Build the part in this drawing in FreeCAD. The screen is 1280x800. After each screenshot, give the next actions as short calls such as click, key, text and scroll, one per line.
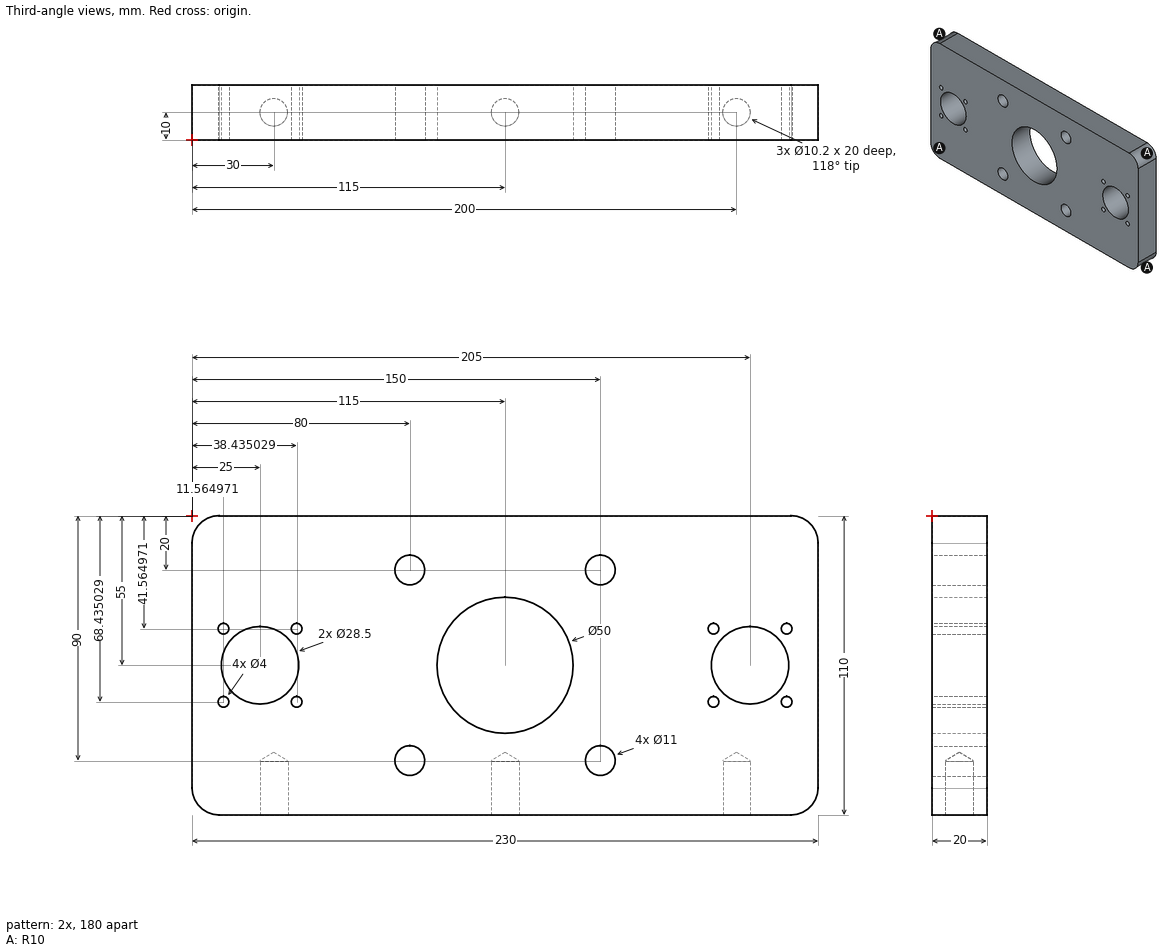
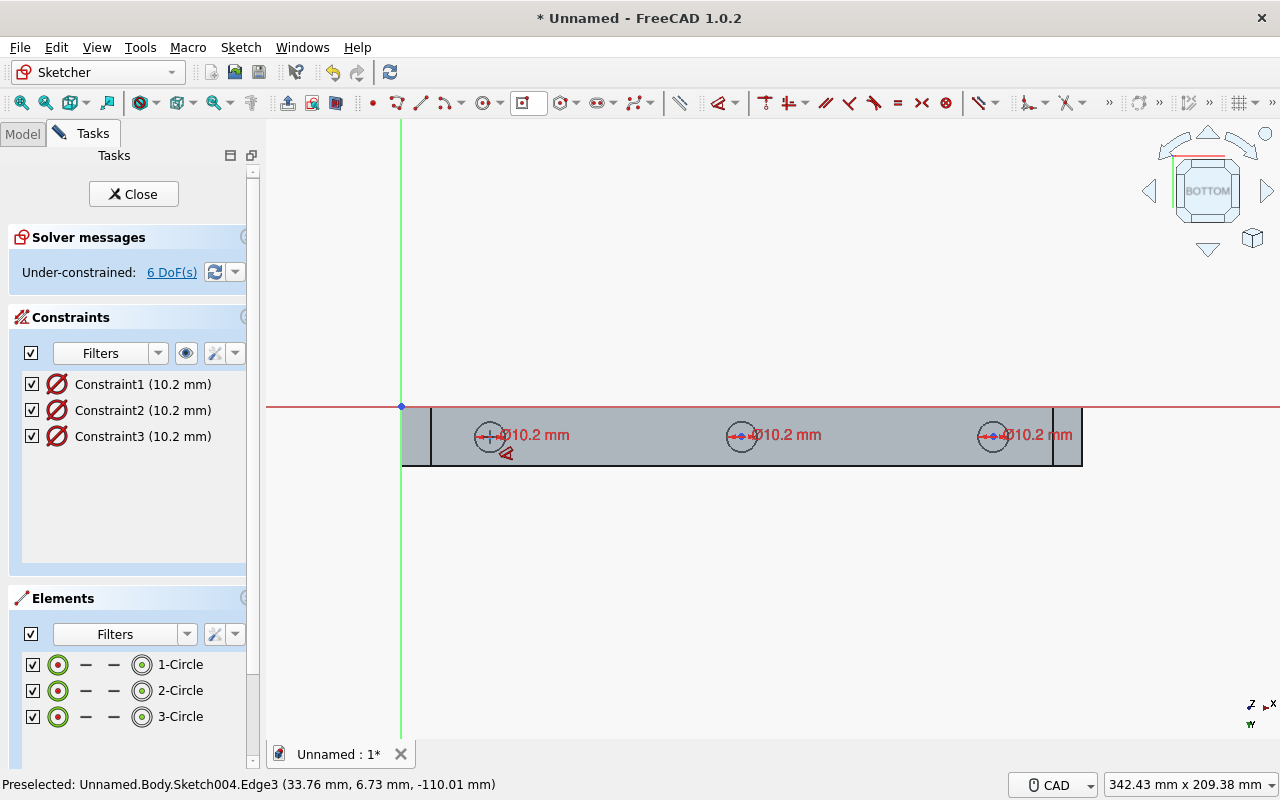
scroll(993, 437, up, 2)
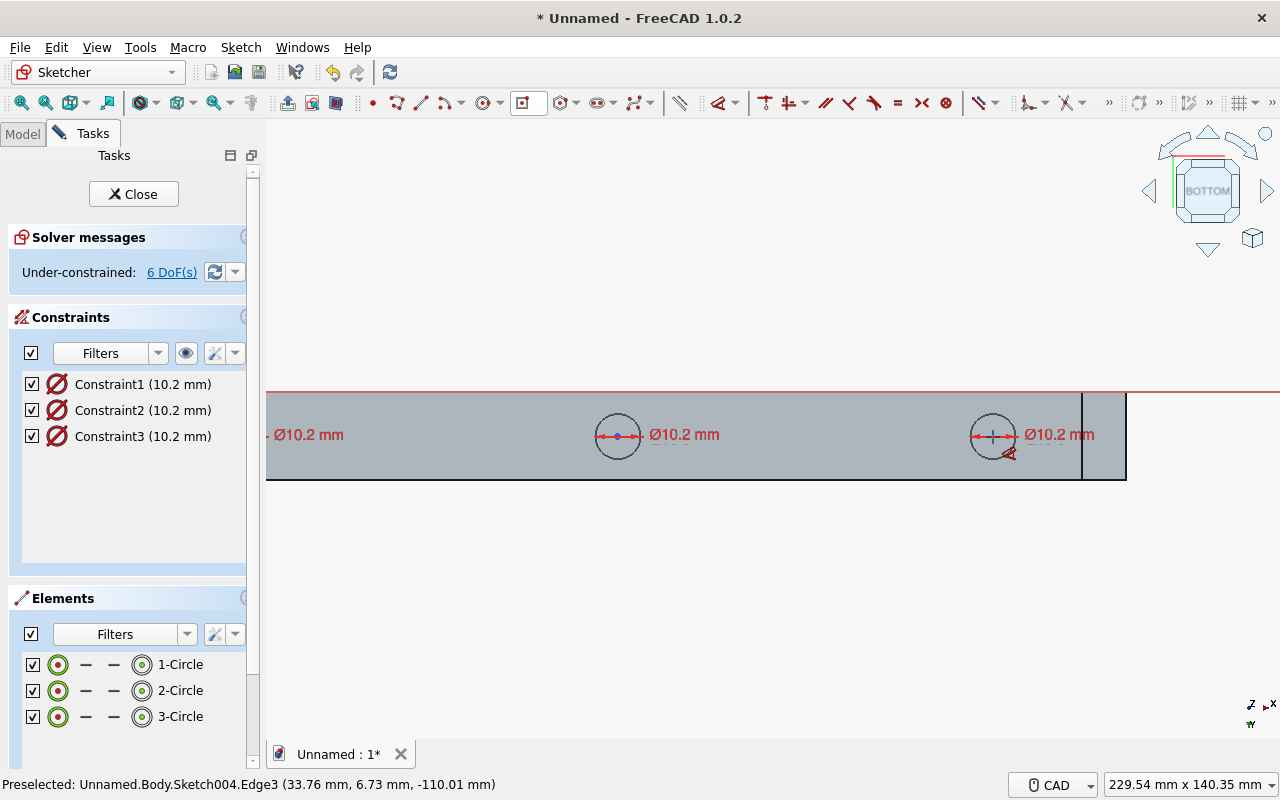
click(993, 437)
click(1027, 414)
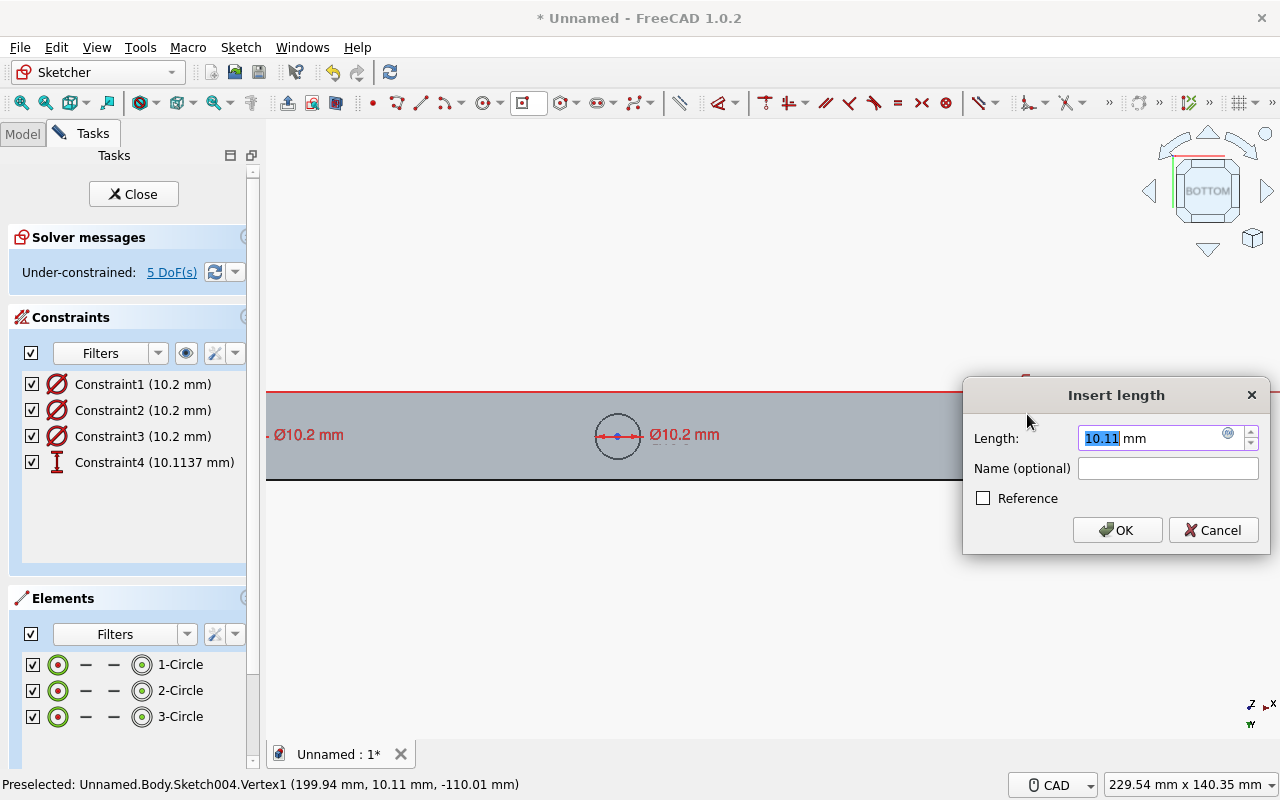
text(10)
key(Return)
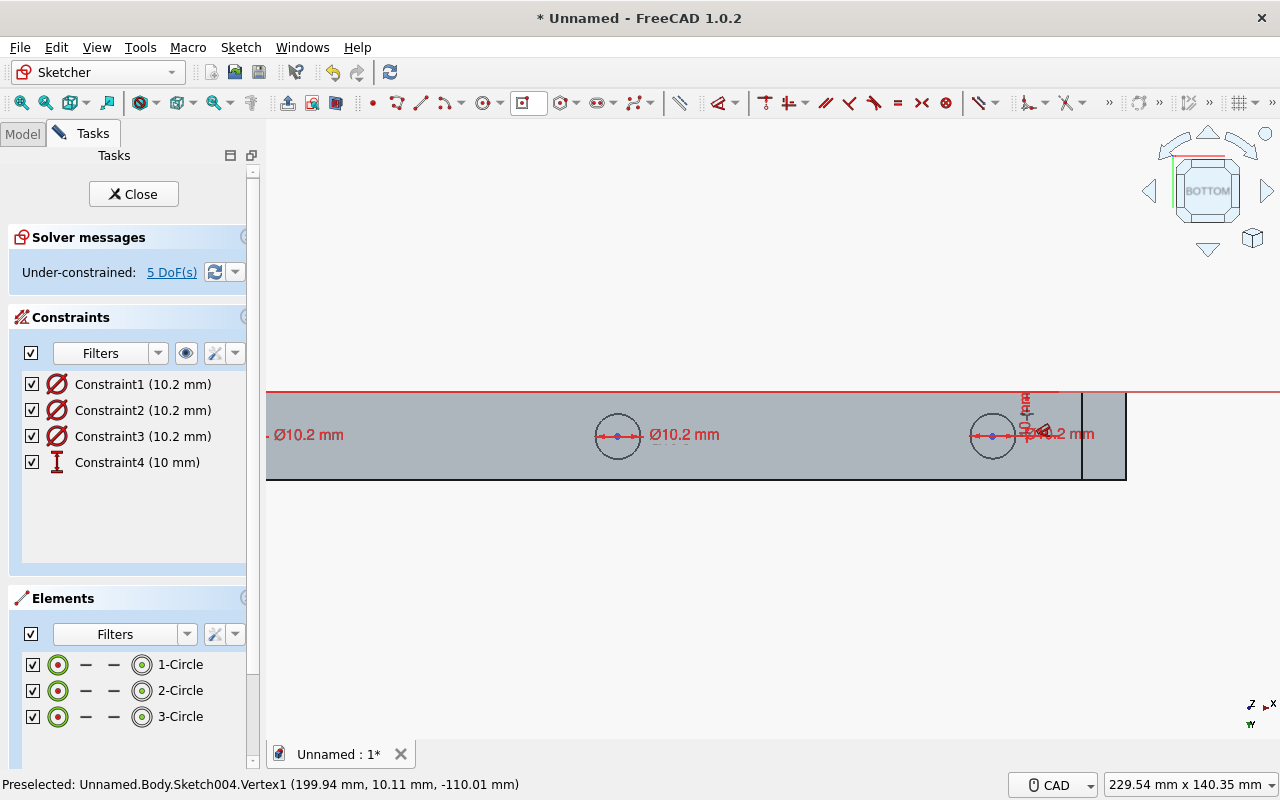
click(618, 437)
click(652, 414)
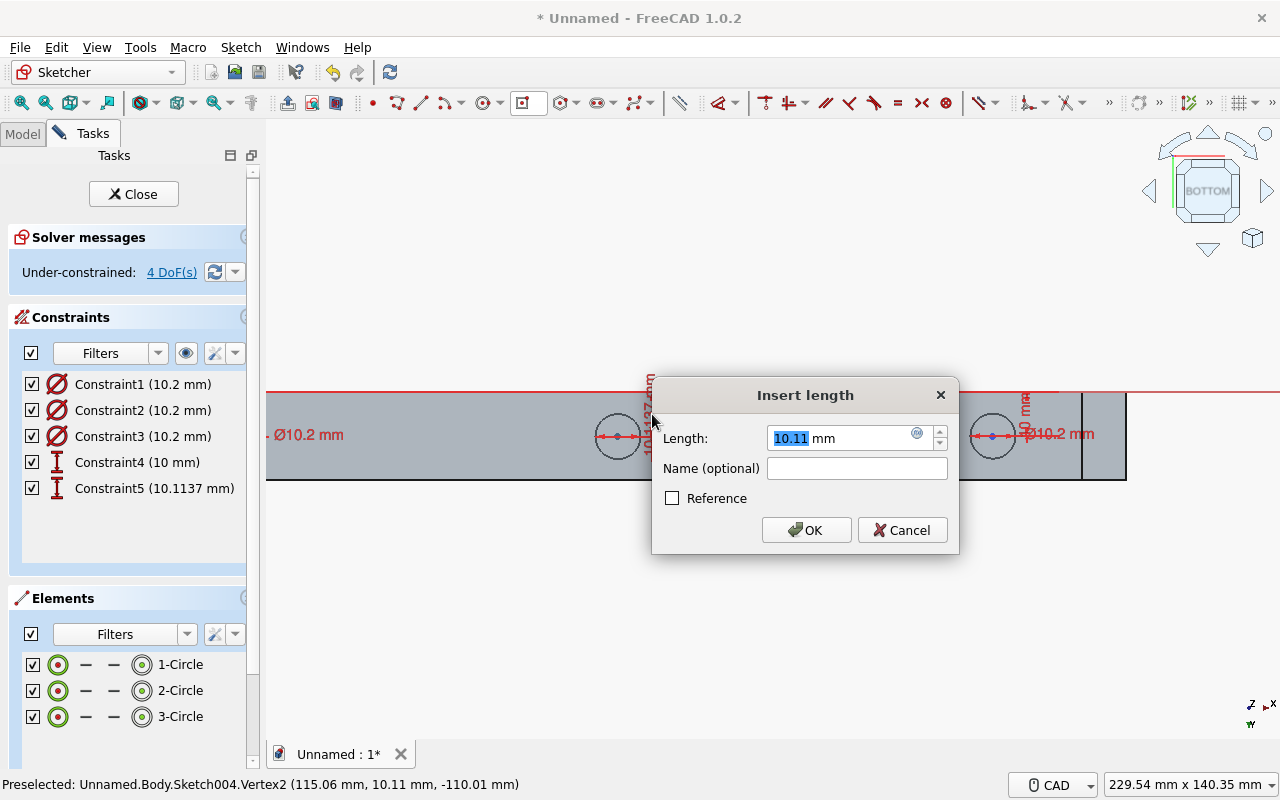
text(10)
key(Return)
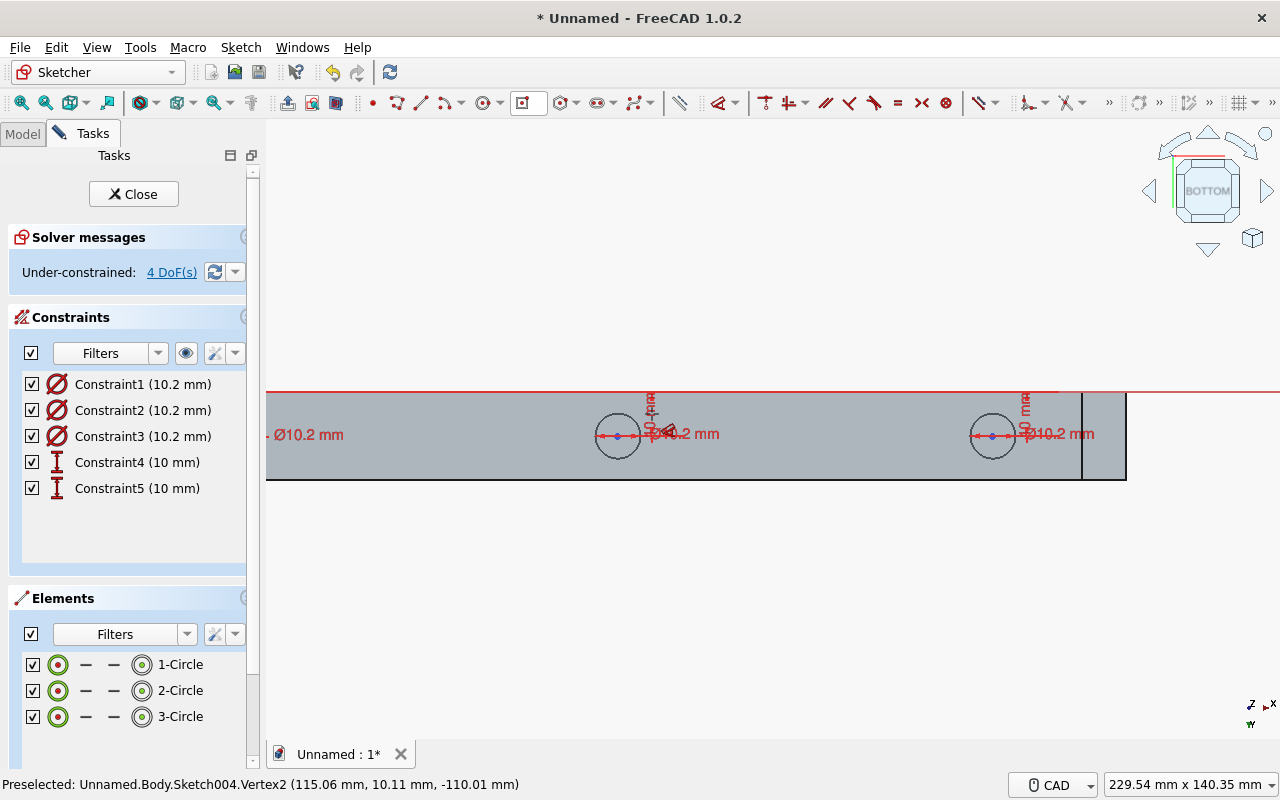
scroll(993, 437, down, 2)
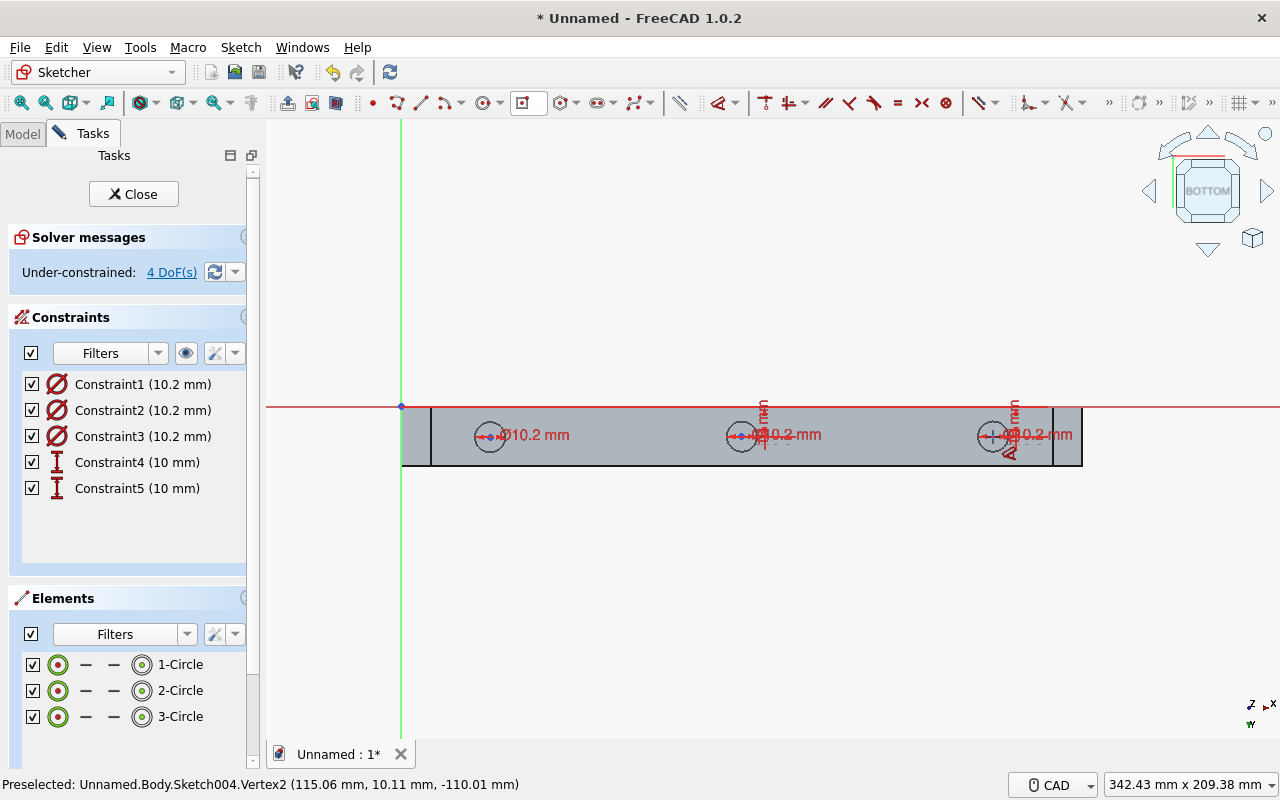
click(490, 437)
click(446, 373)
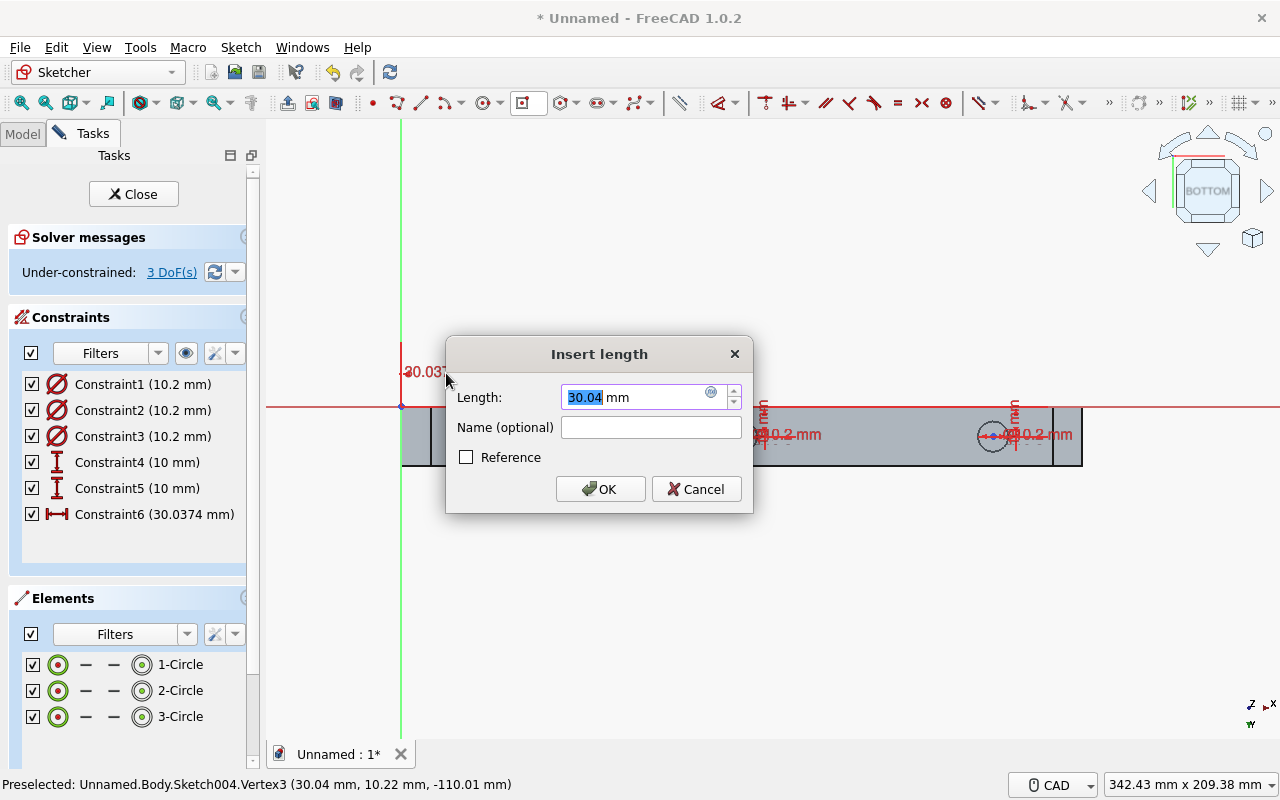
text(30)
key(Return)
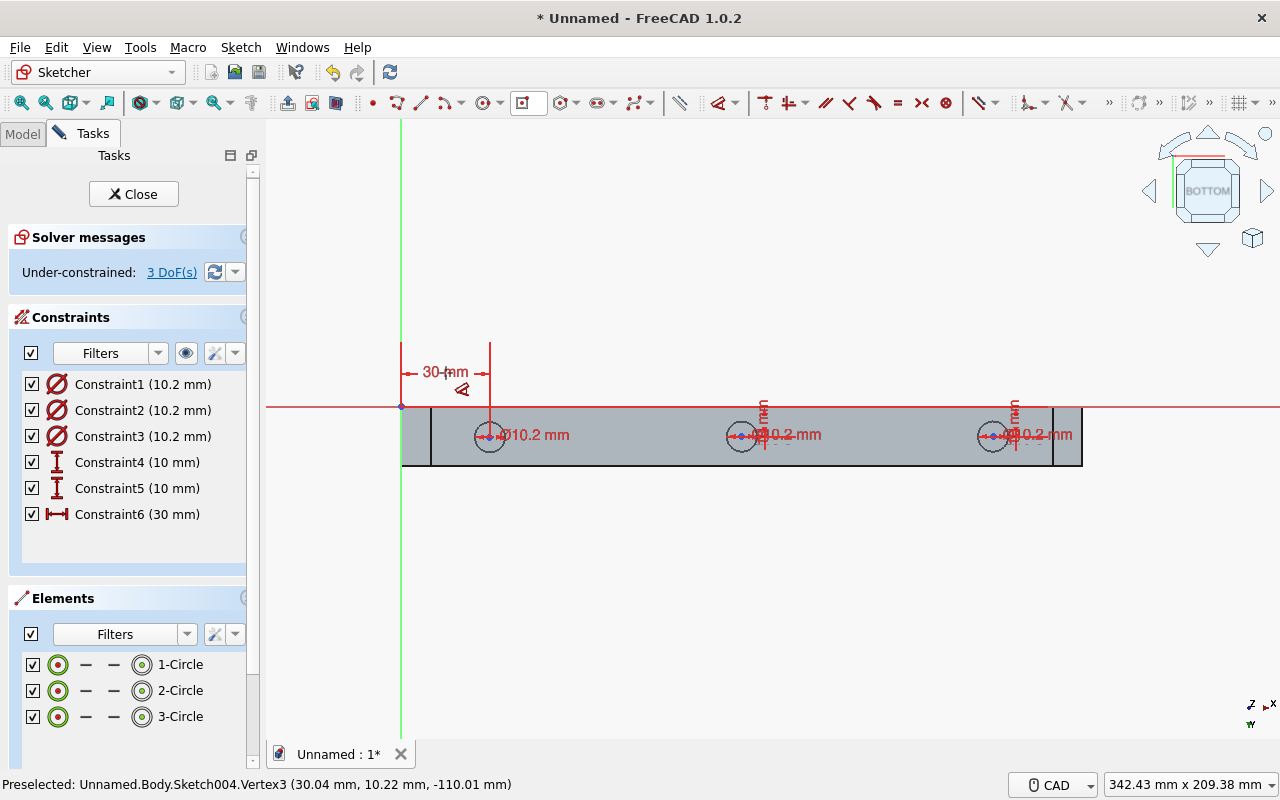
scroll(490, 437, up, 2)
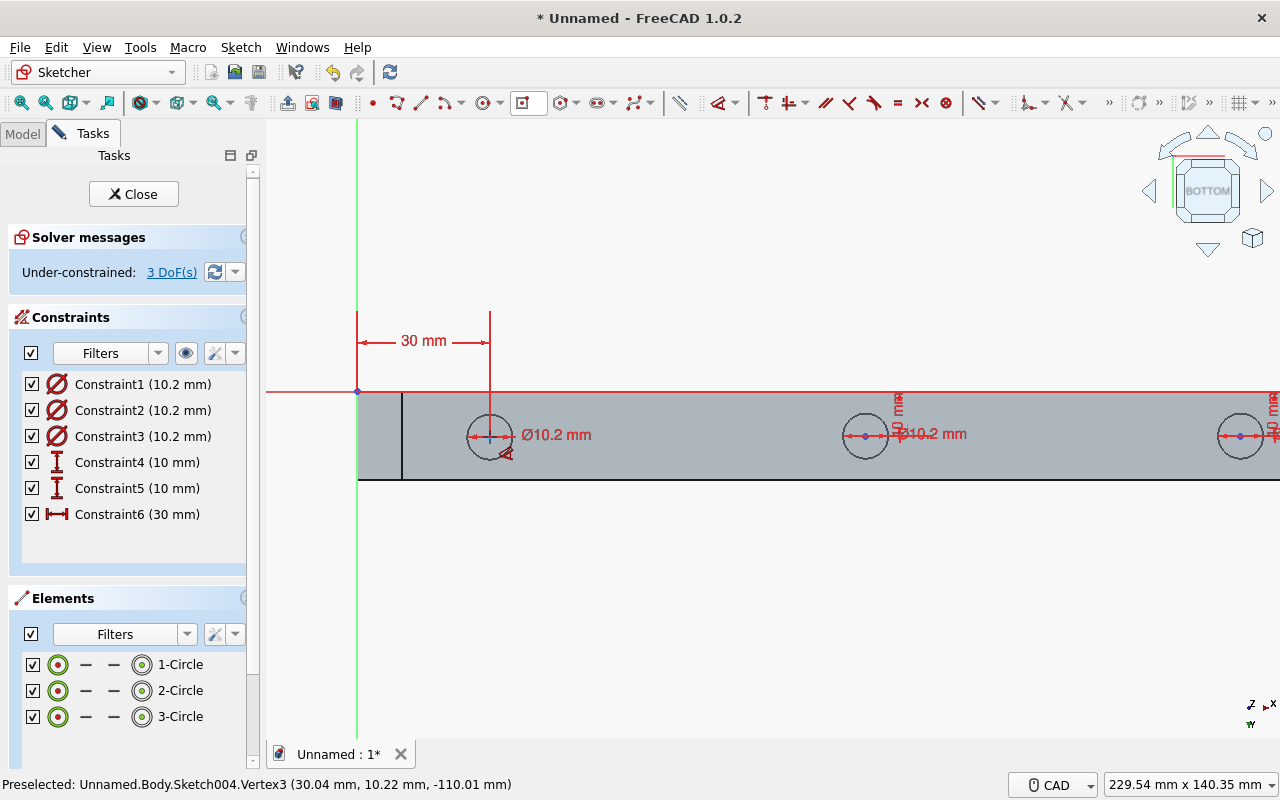
click(490, 437)
click(323, 415)